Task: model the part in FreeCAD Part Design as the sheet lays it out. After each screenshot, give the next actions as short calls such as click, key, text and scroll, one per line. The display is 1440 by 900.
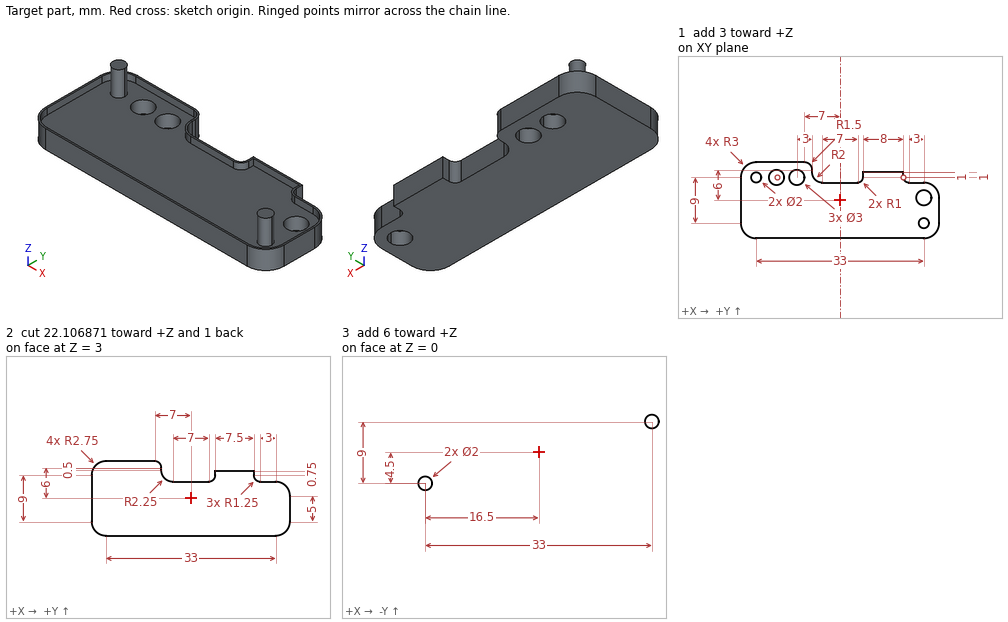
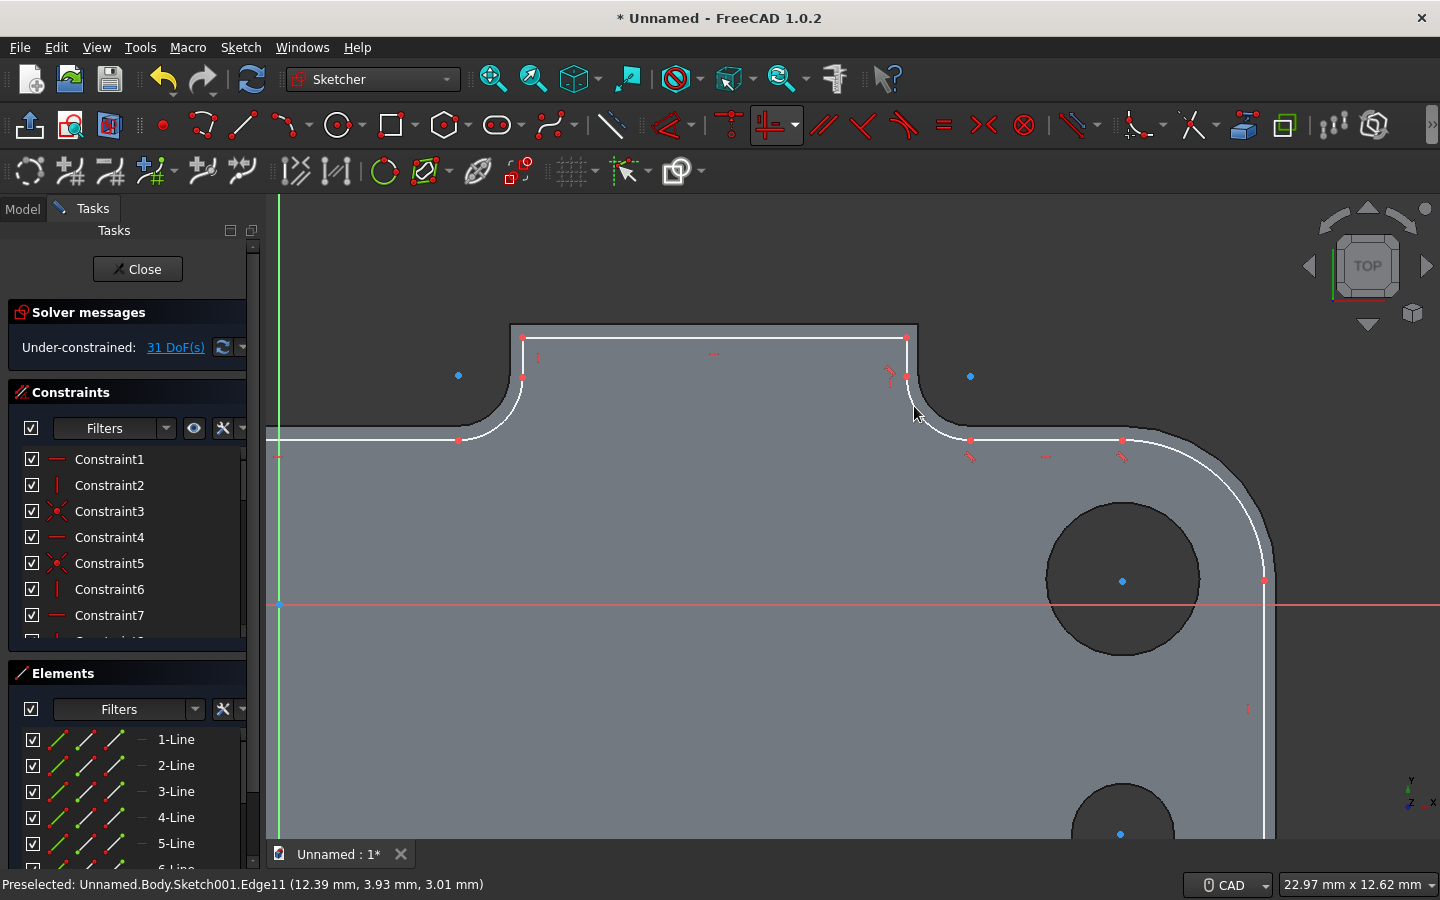
click(523, 350)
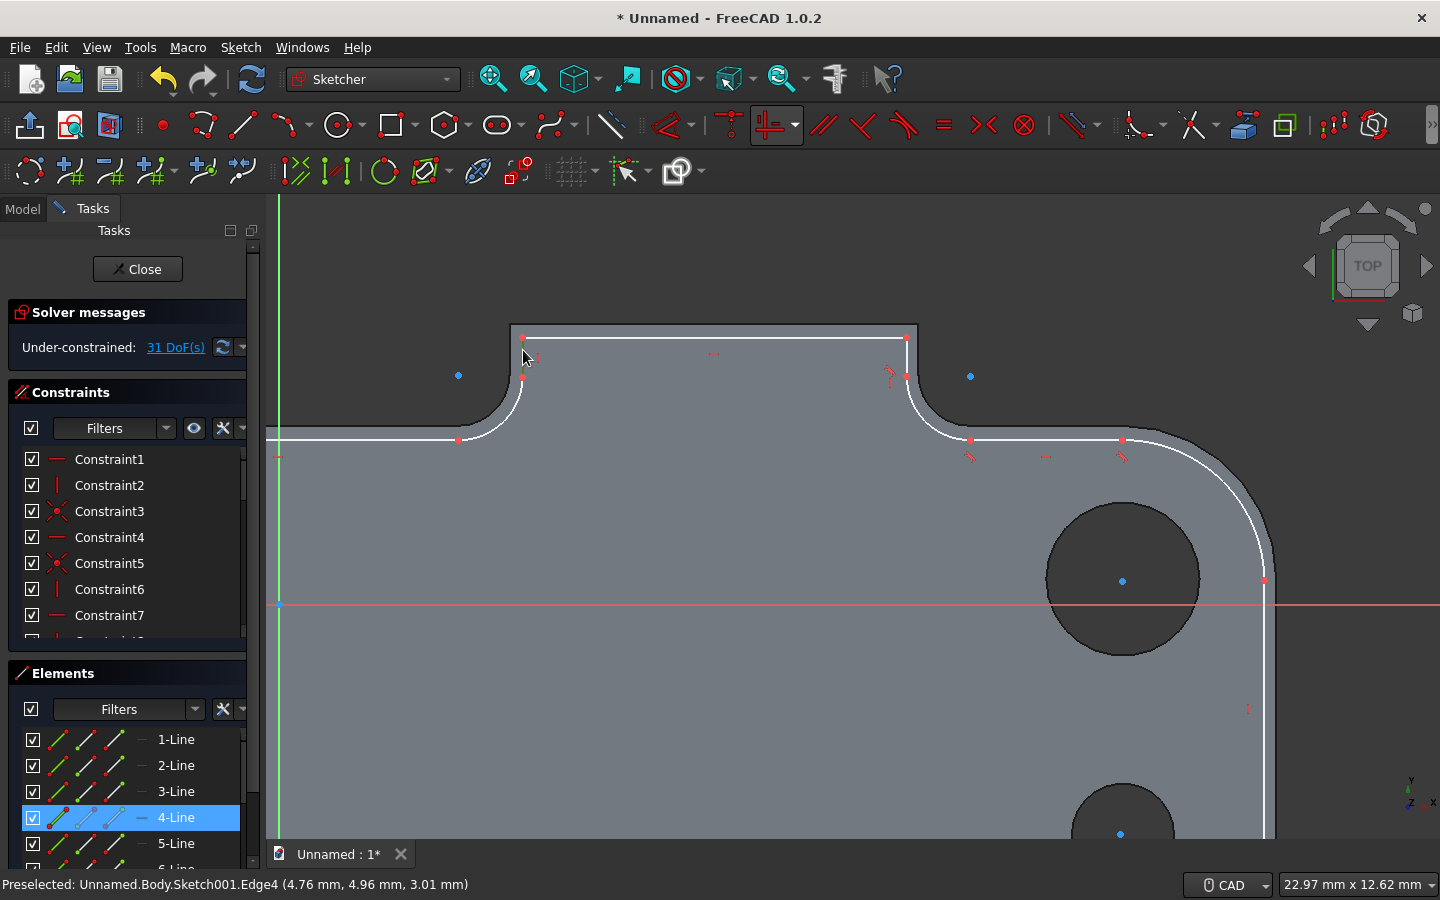
click(487, 434)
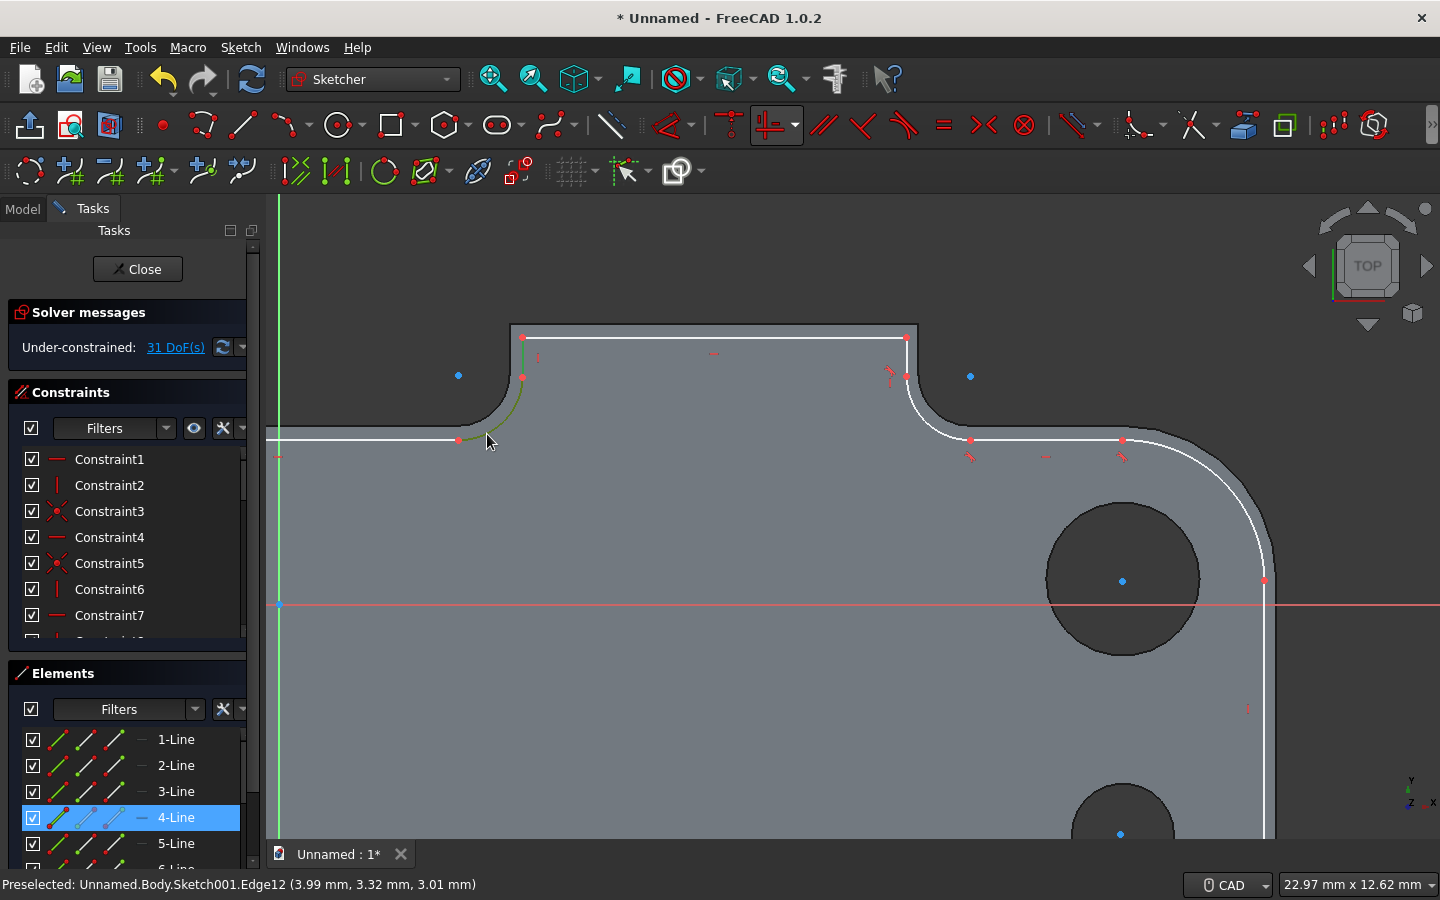
click(904, 126)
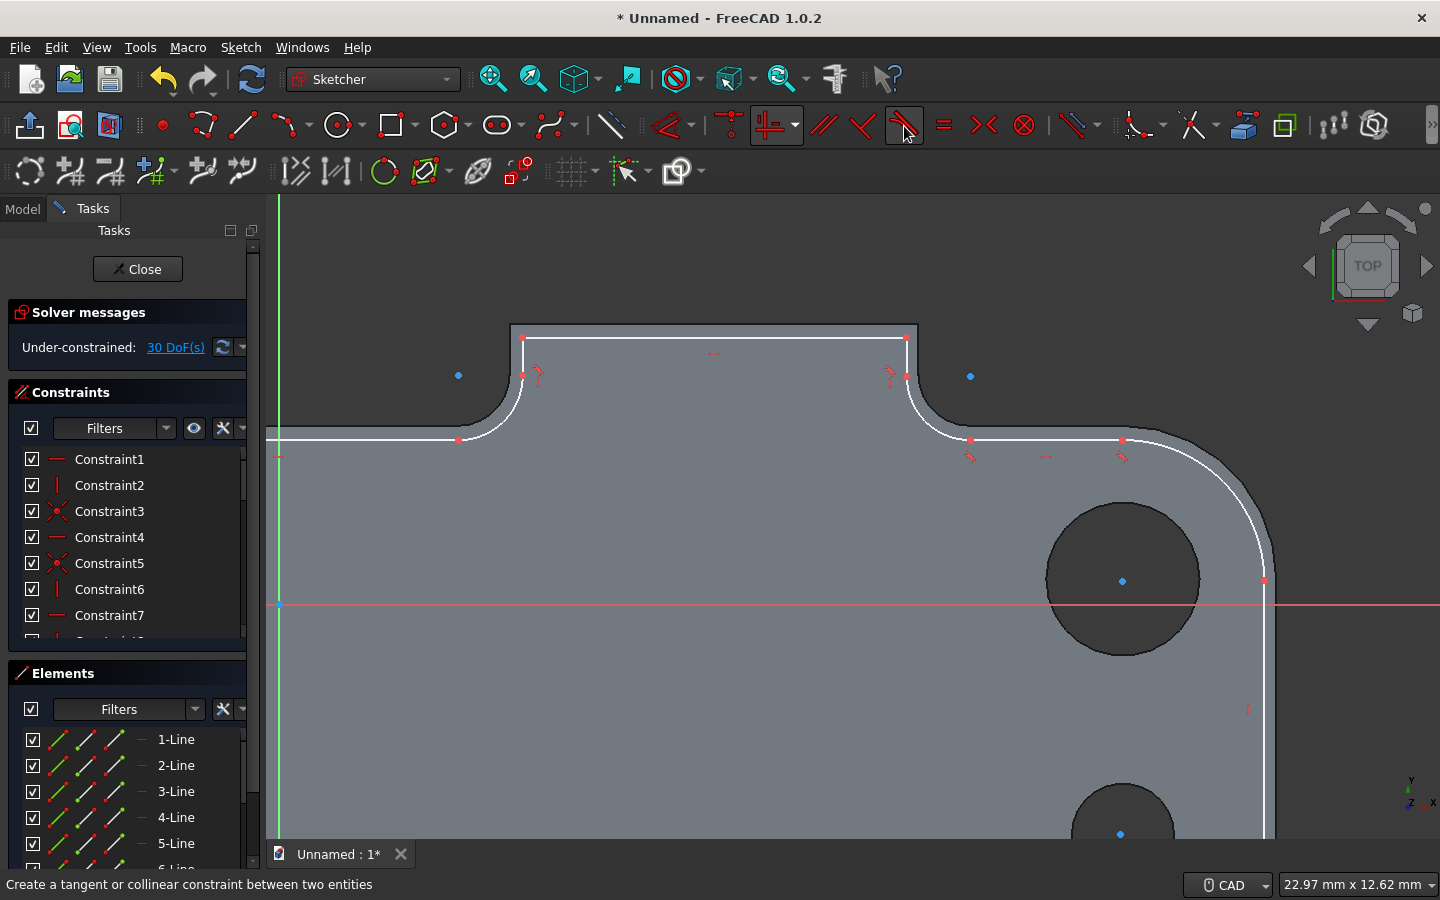
click(351, 440)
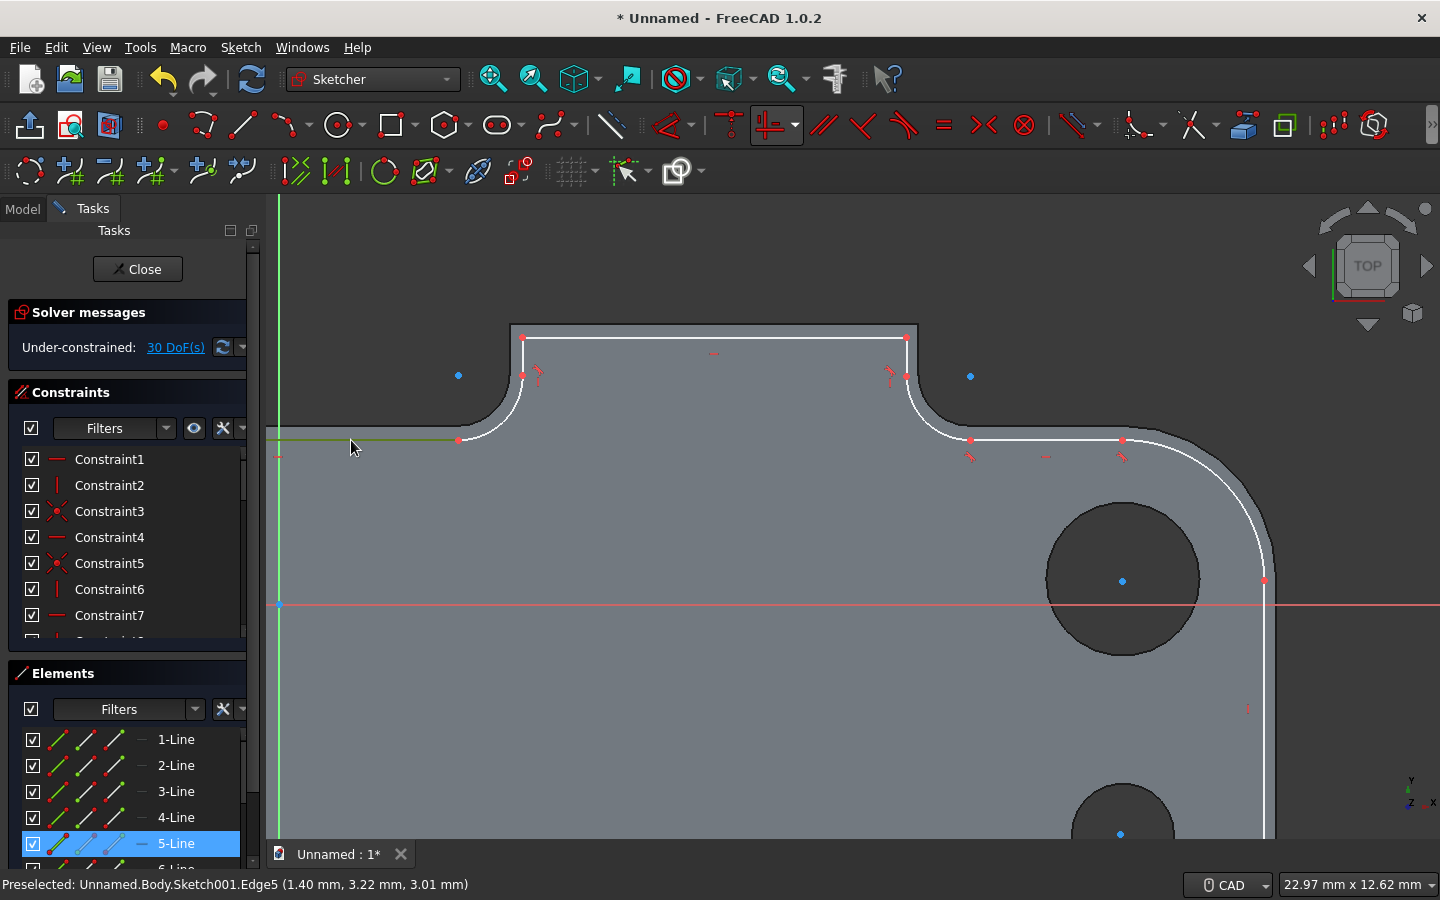
click(487, 433)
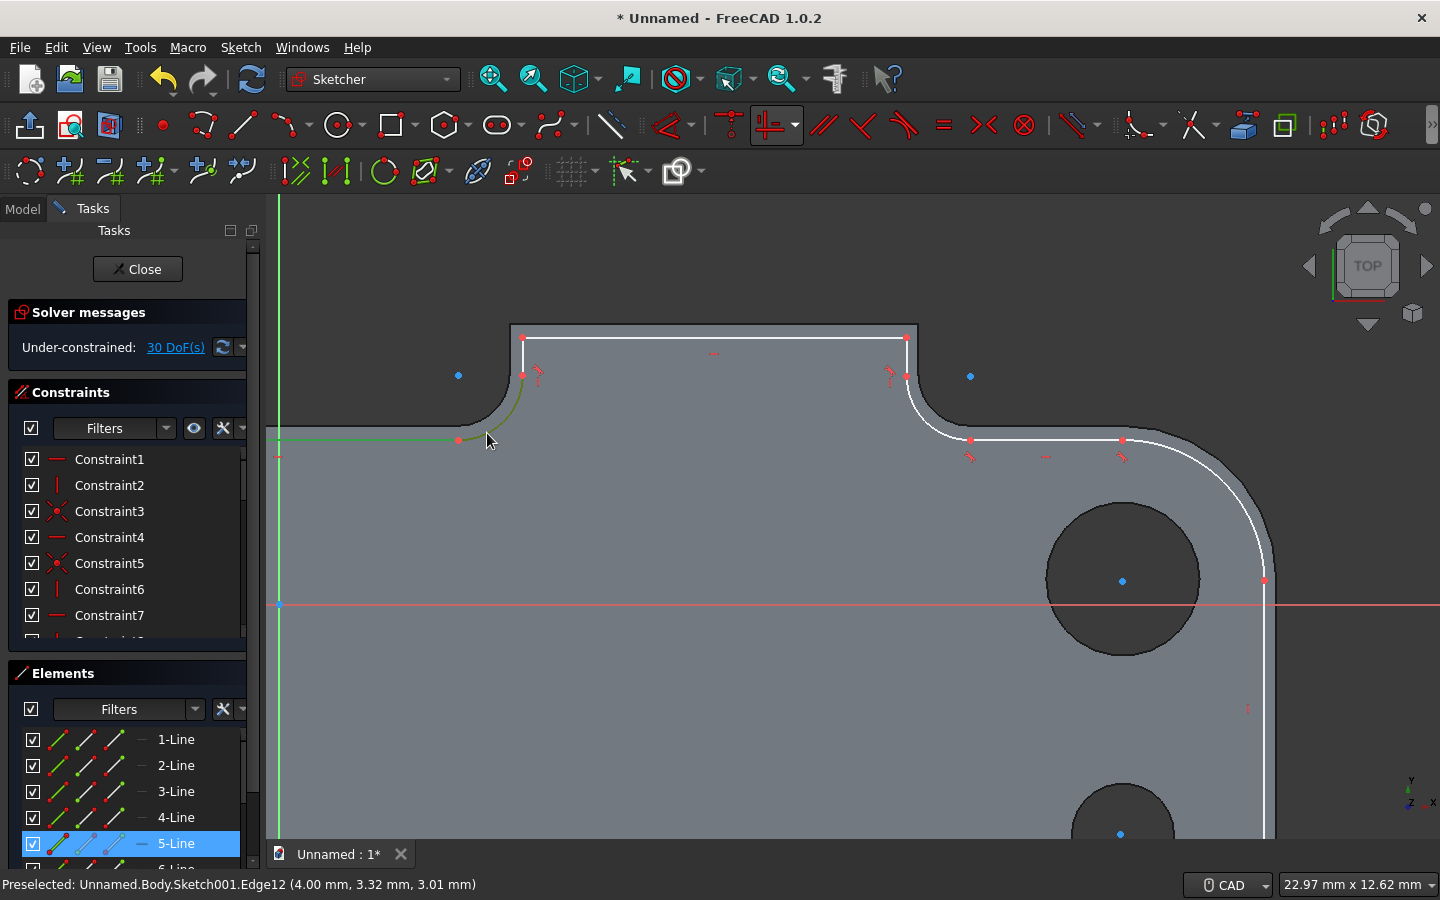
click(904, 126)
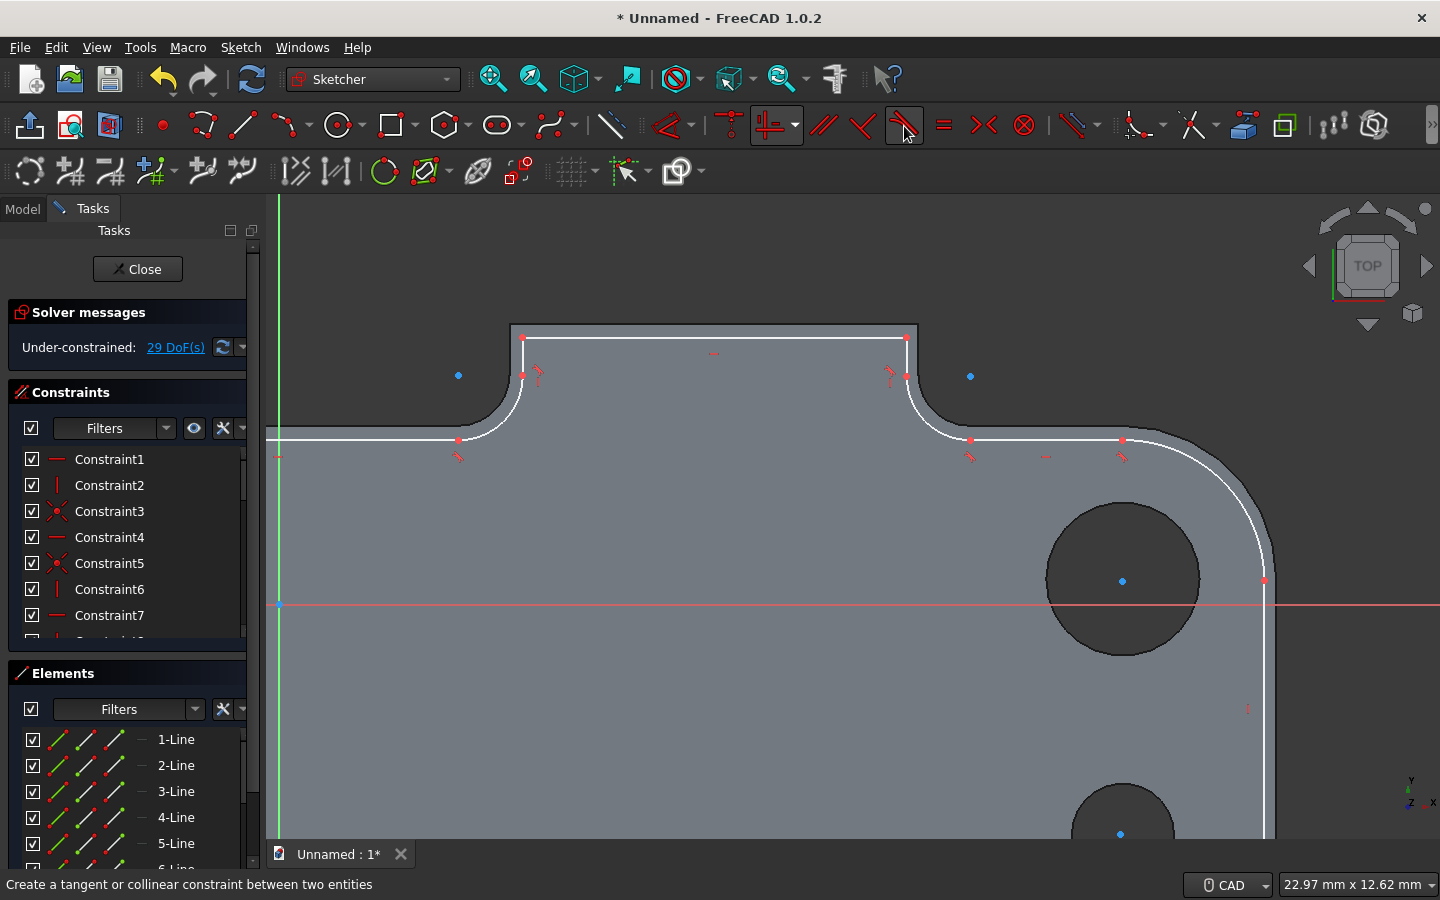
click(351, 440)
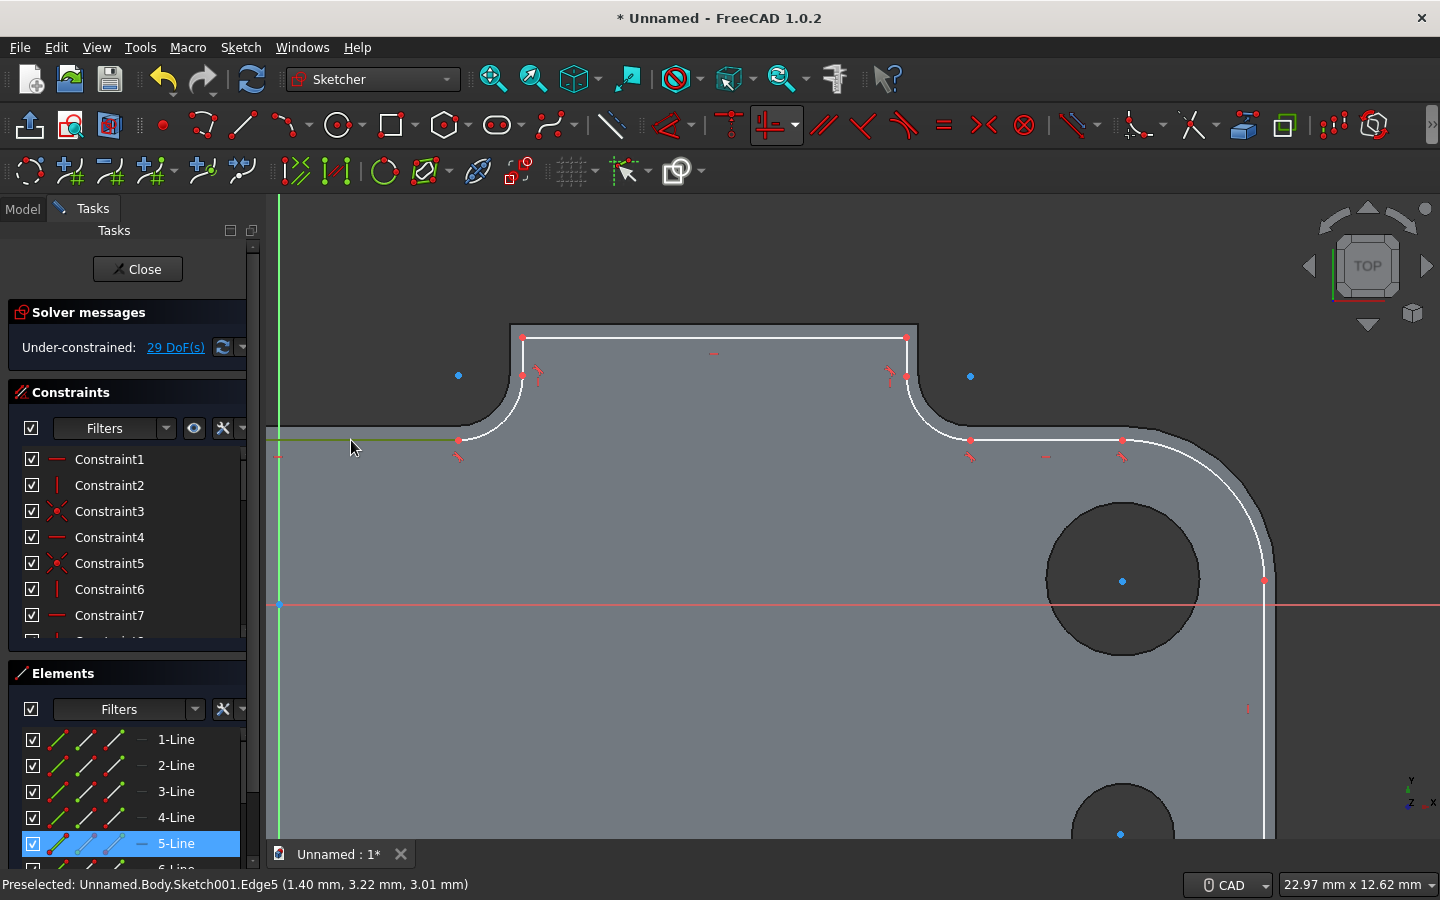
scroll(1078, 465, down, 5)